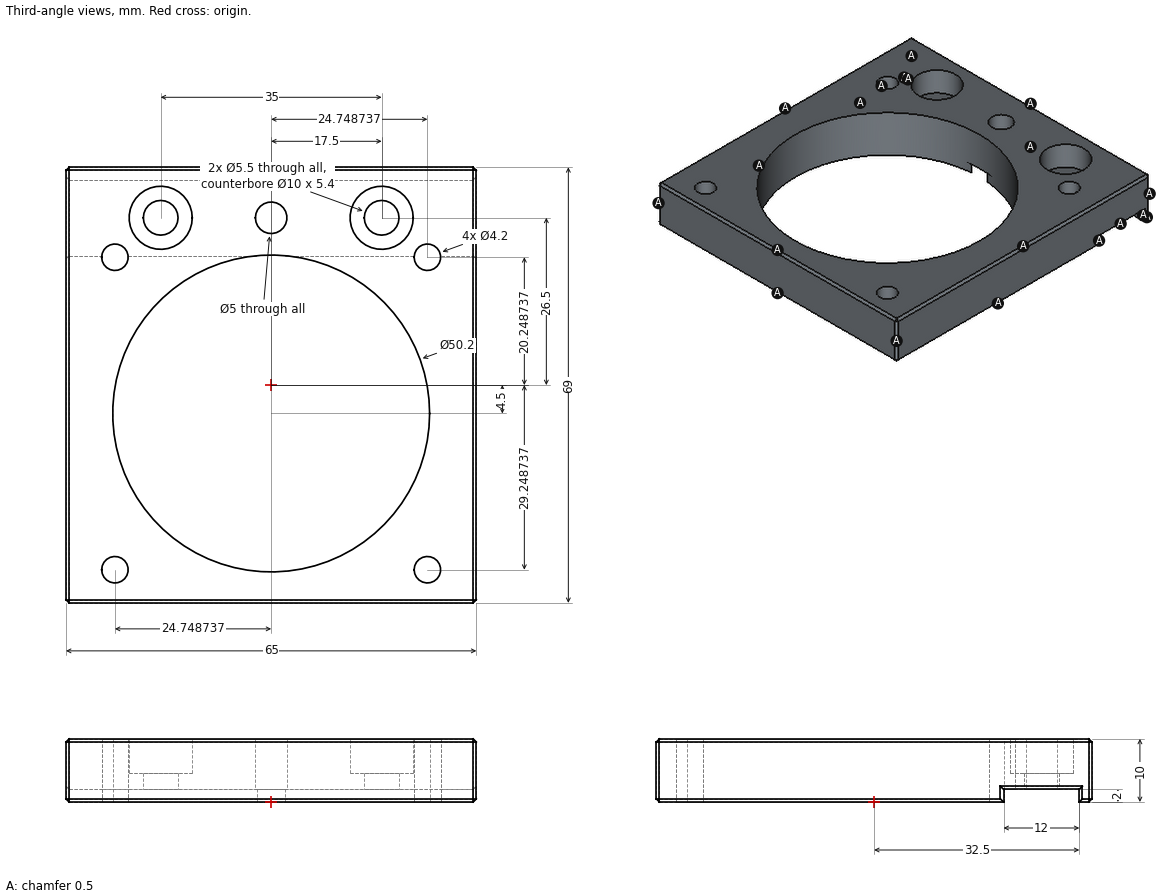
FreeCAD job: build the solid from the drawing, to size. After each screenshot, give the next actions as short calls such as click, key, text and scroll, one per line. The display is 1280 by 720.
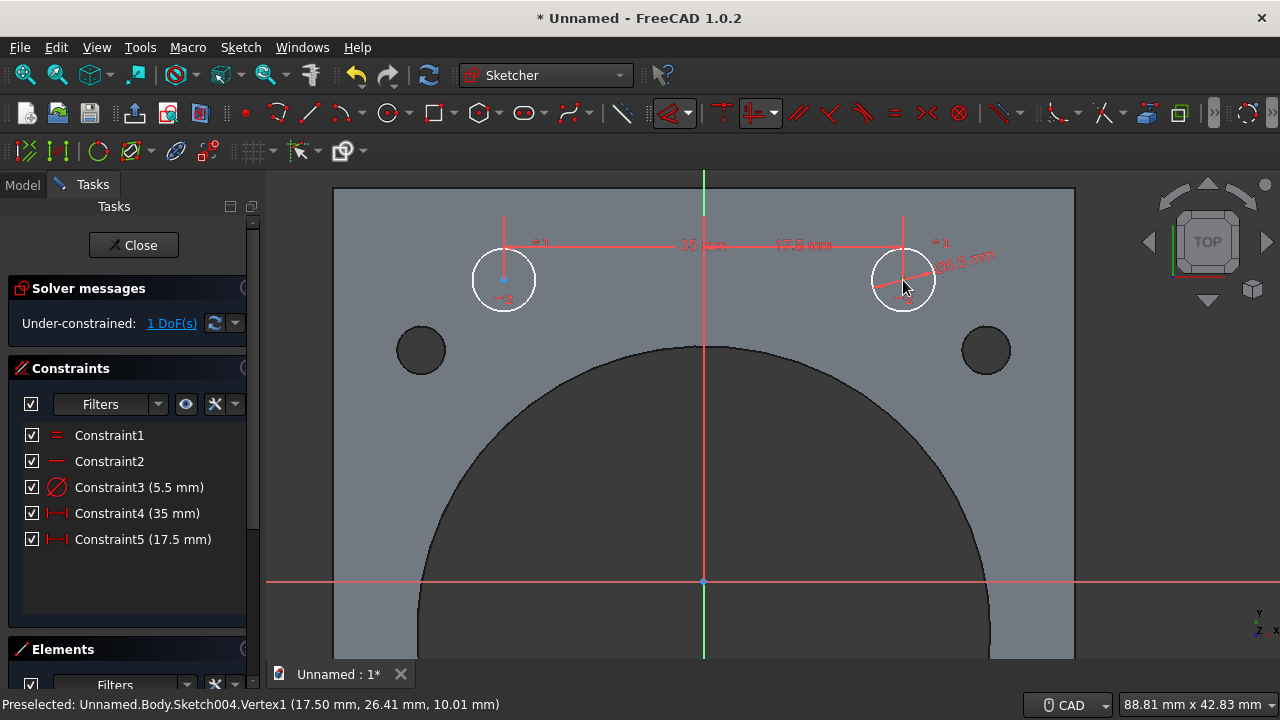
key(i)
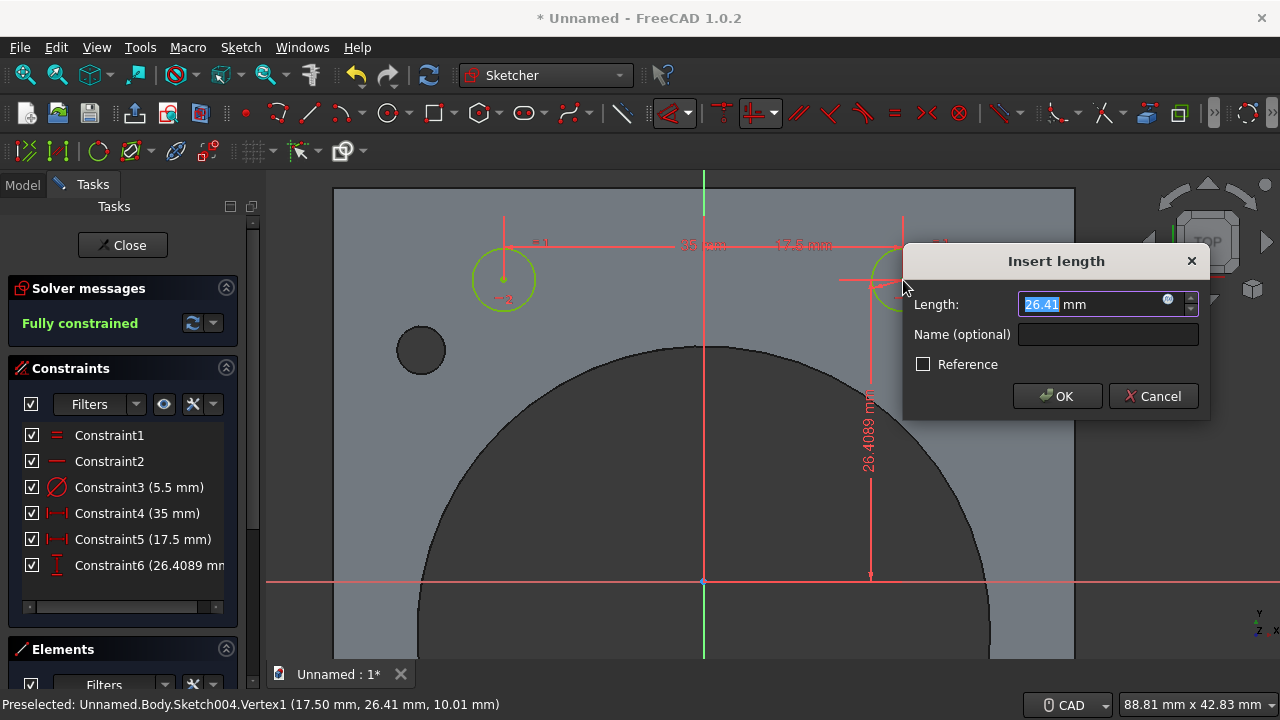
text(26.5)
key(Return)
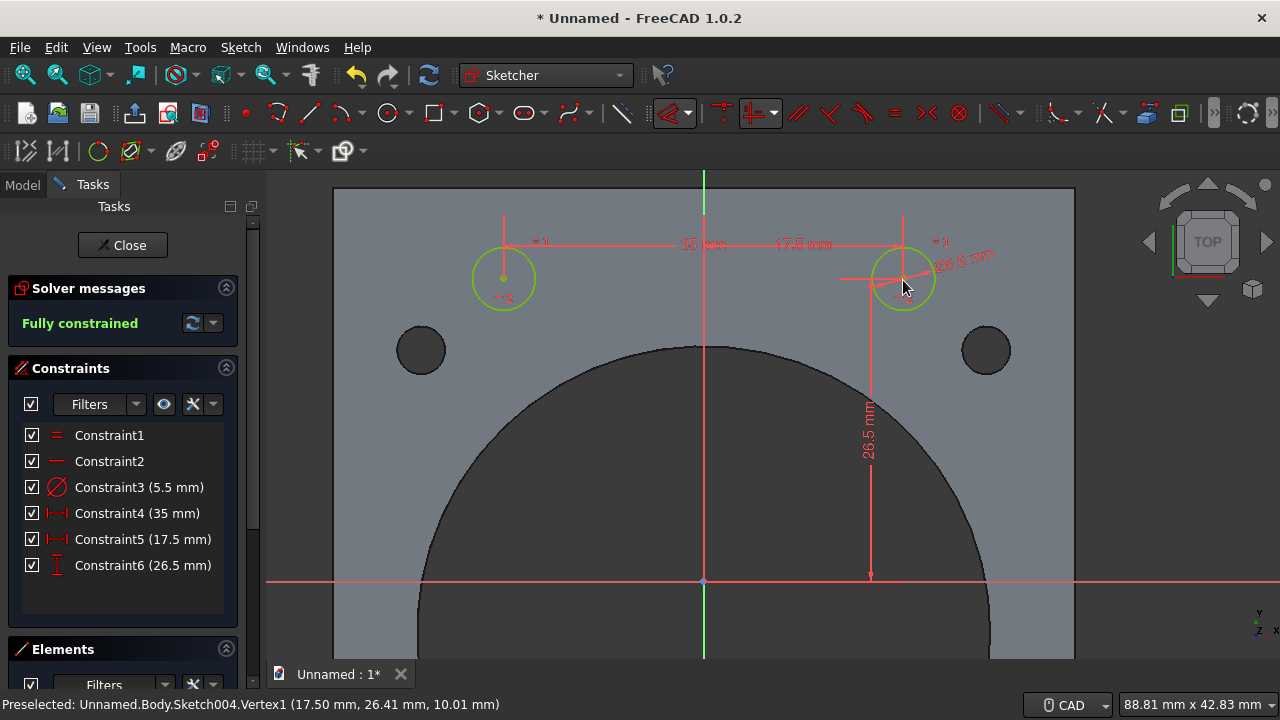
click(123, 245)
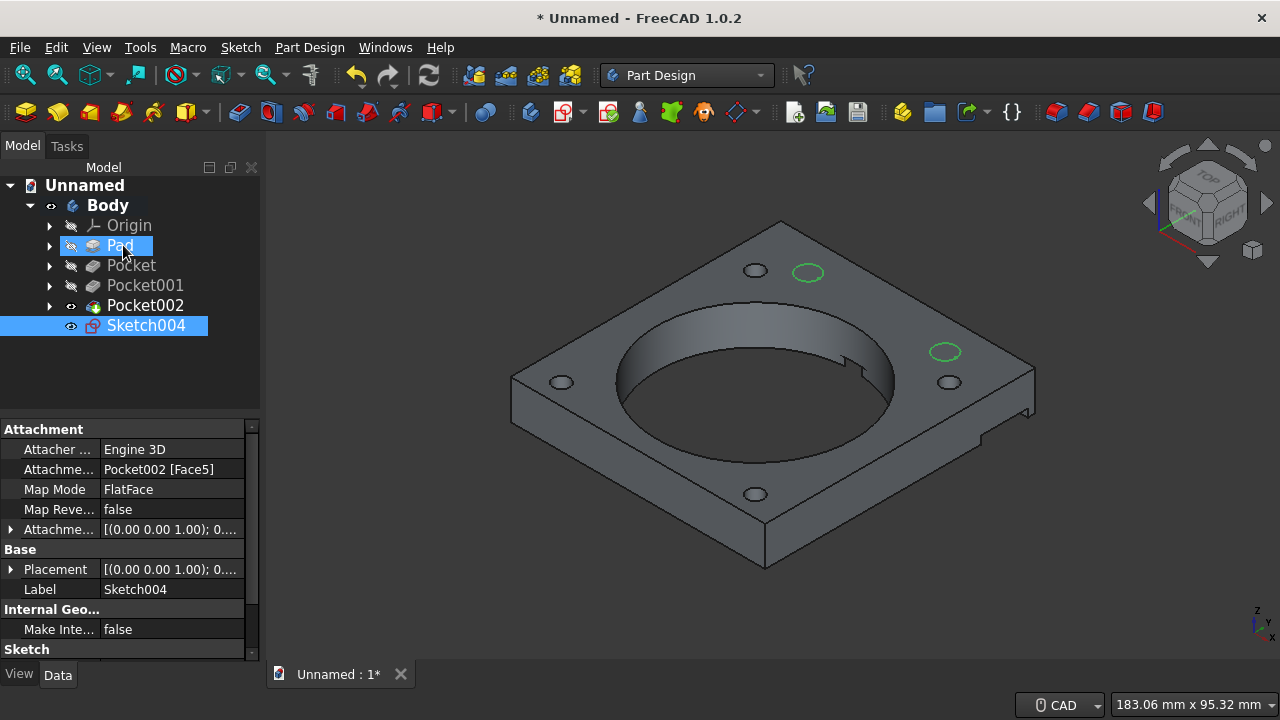
click(272, 112)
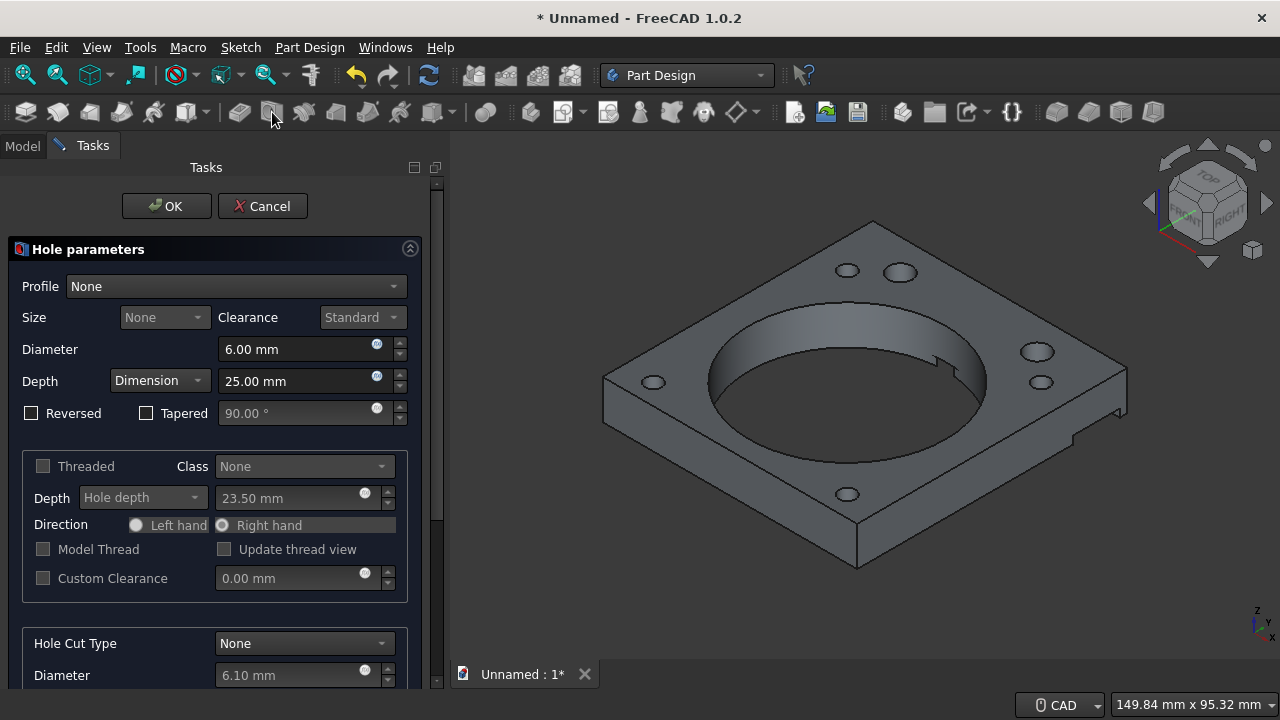
triple_click(305, 349)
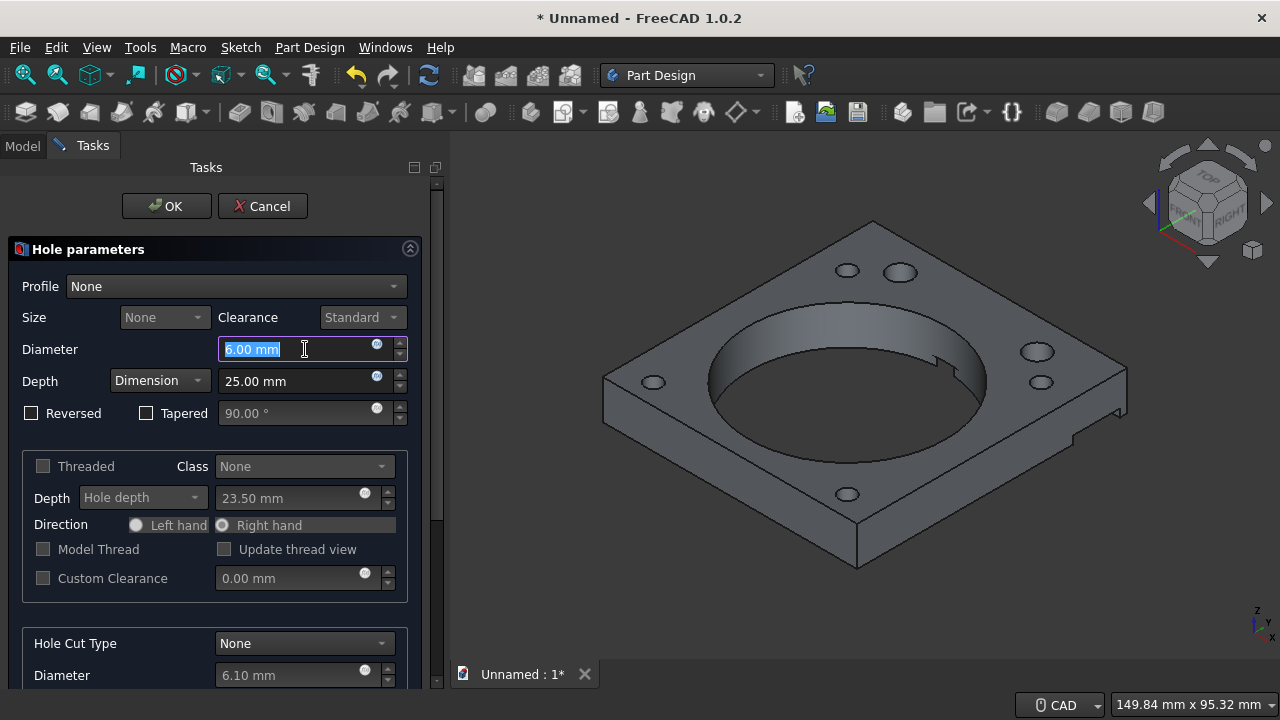
text(5.5)
key(Tab)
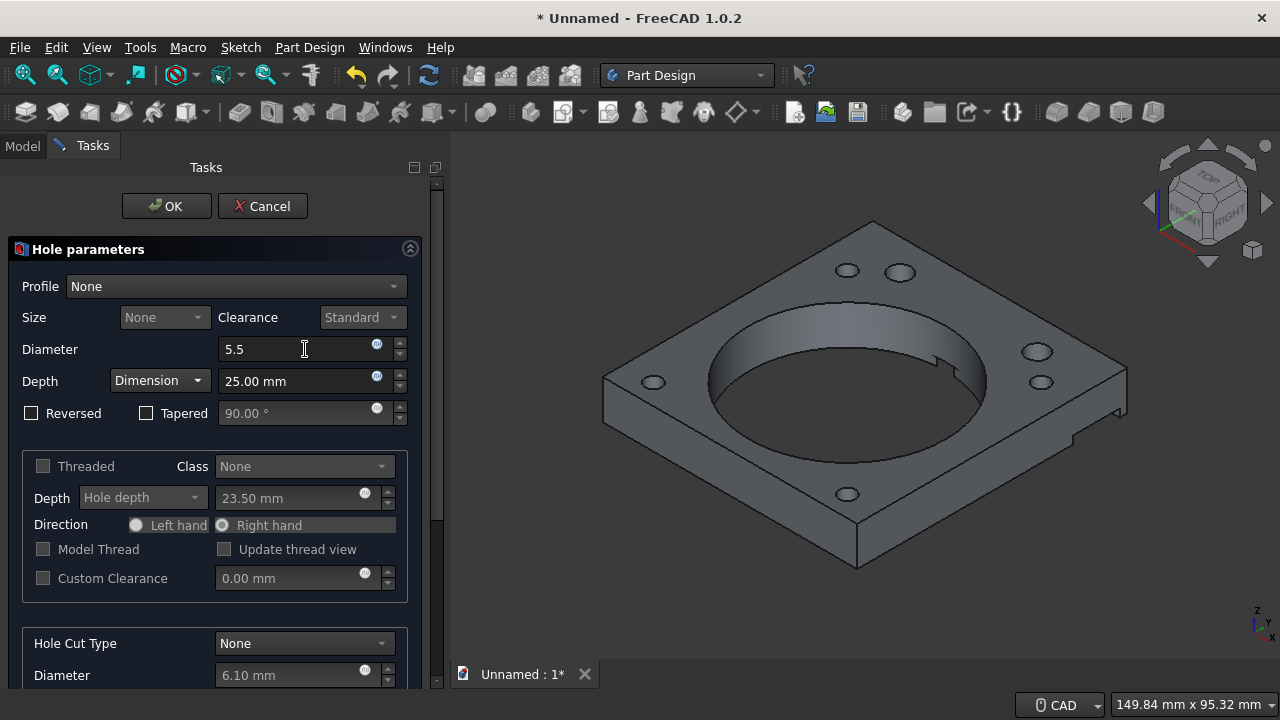
click(161, 380)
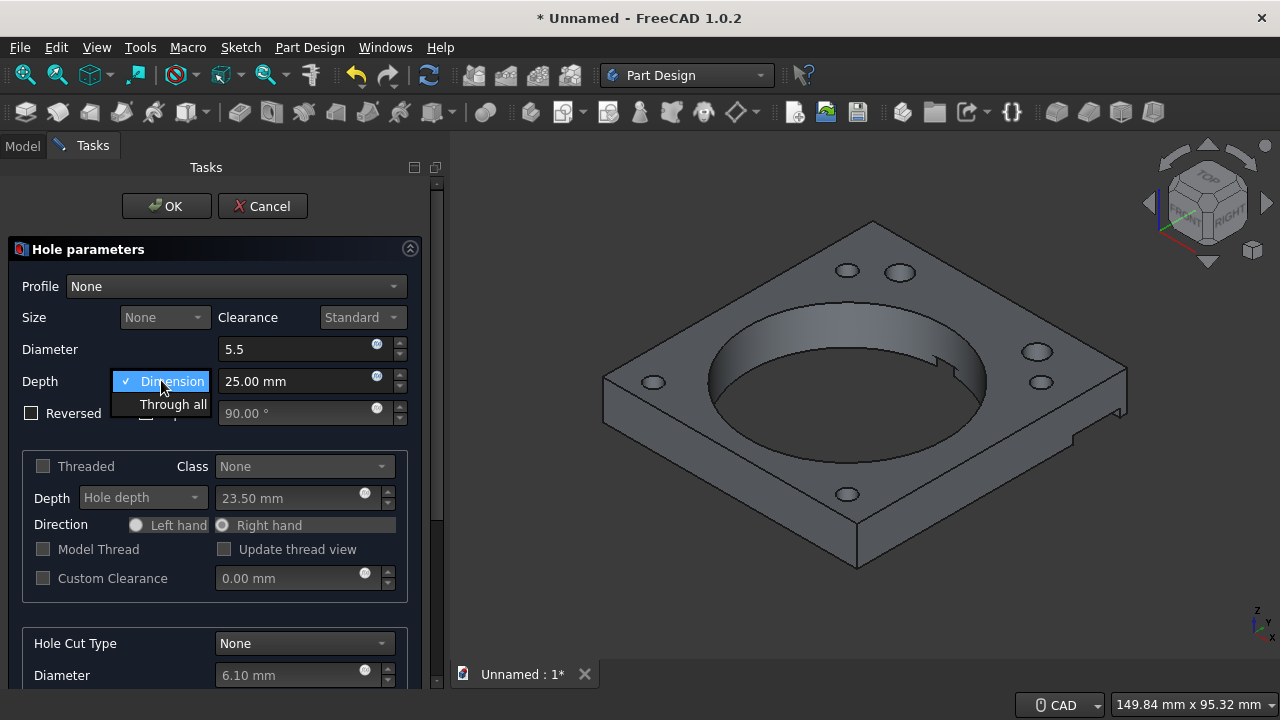
click(160, 404)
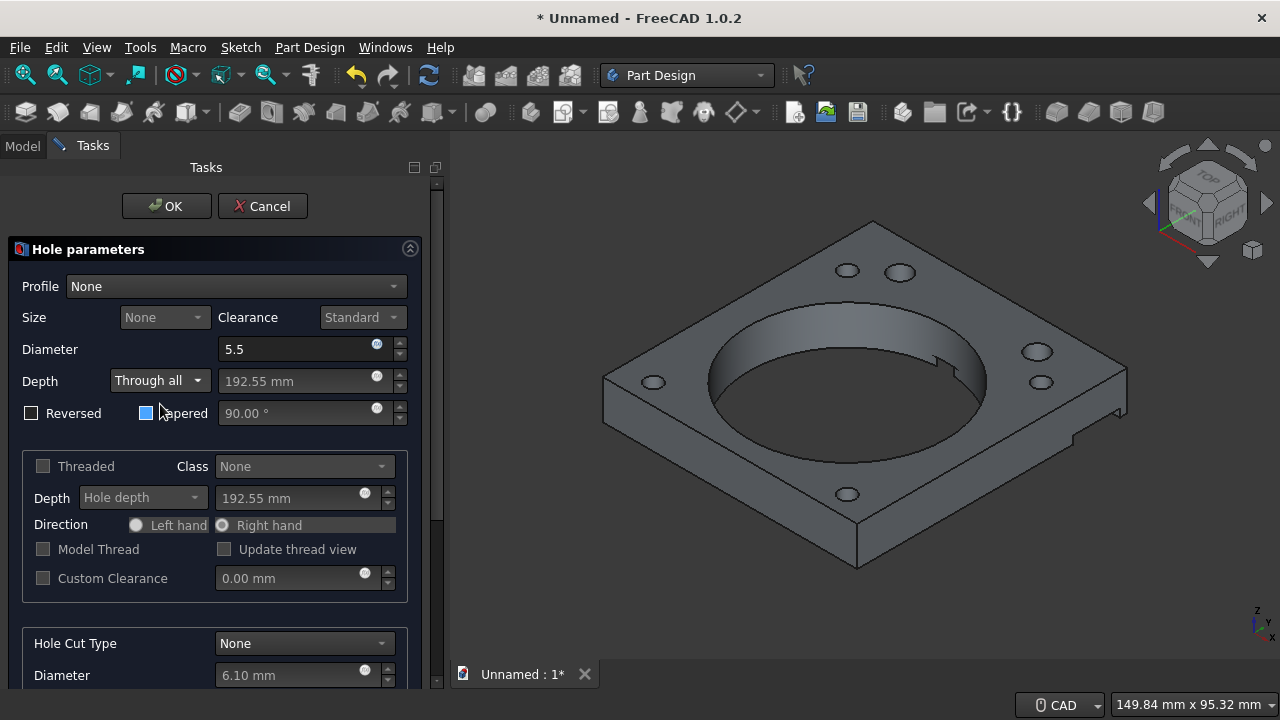
click(306, 644)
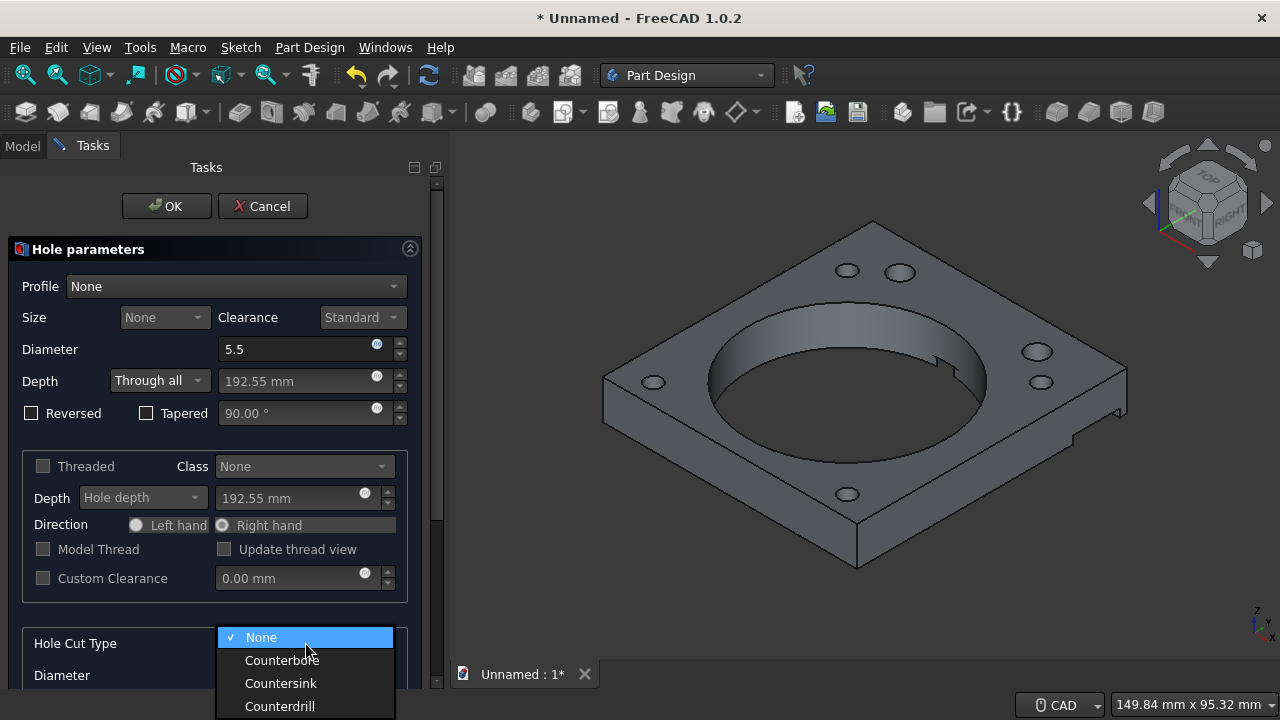
click(304, 660)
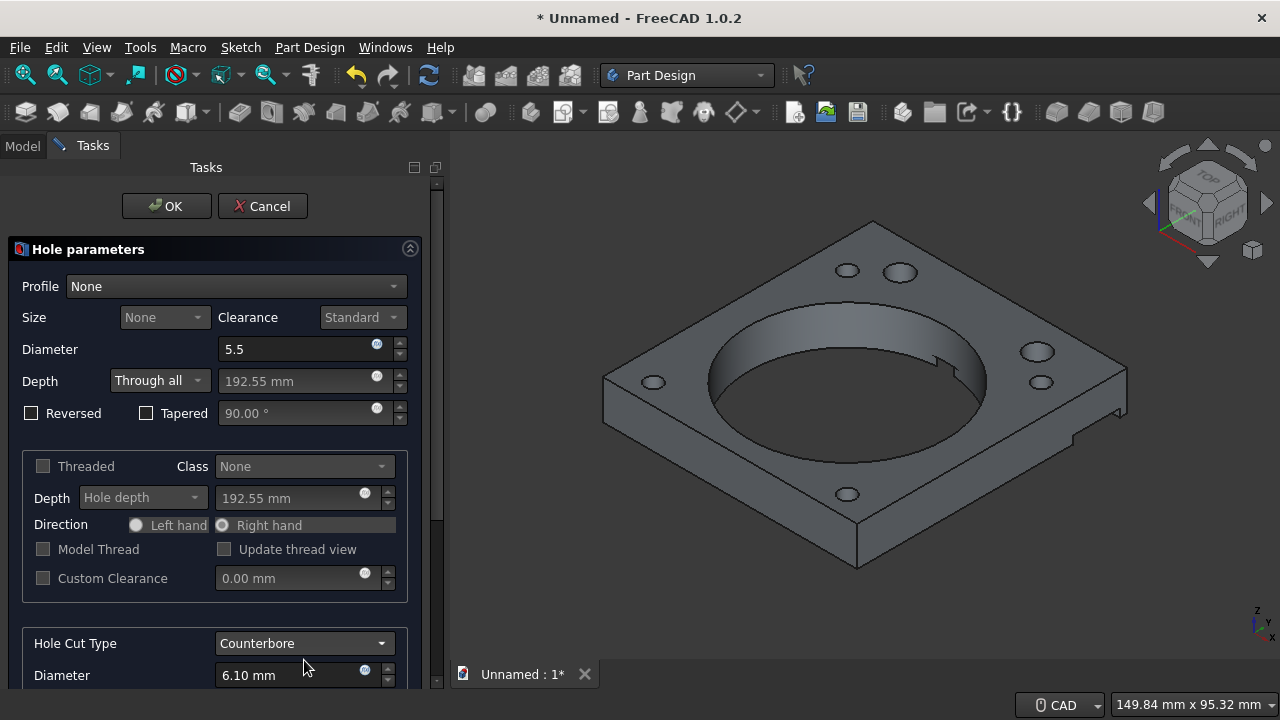
triple_click(298, 675)